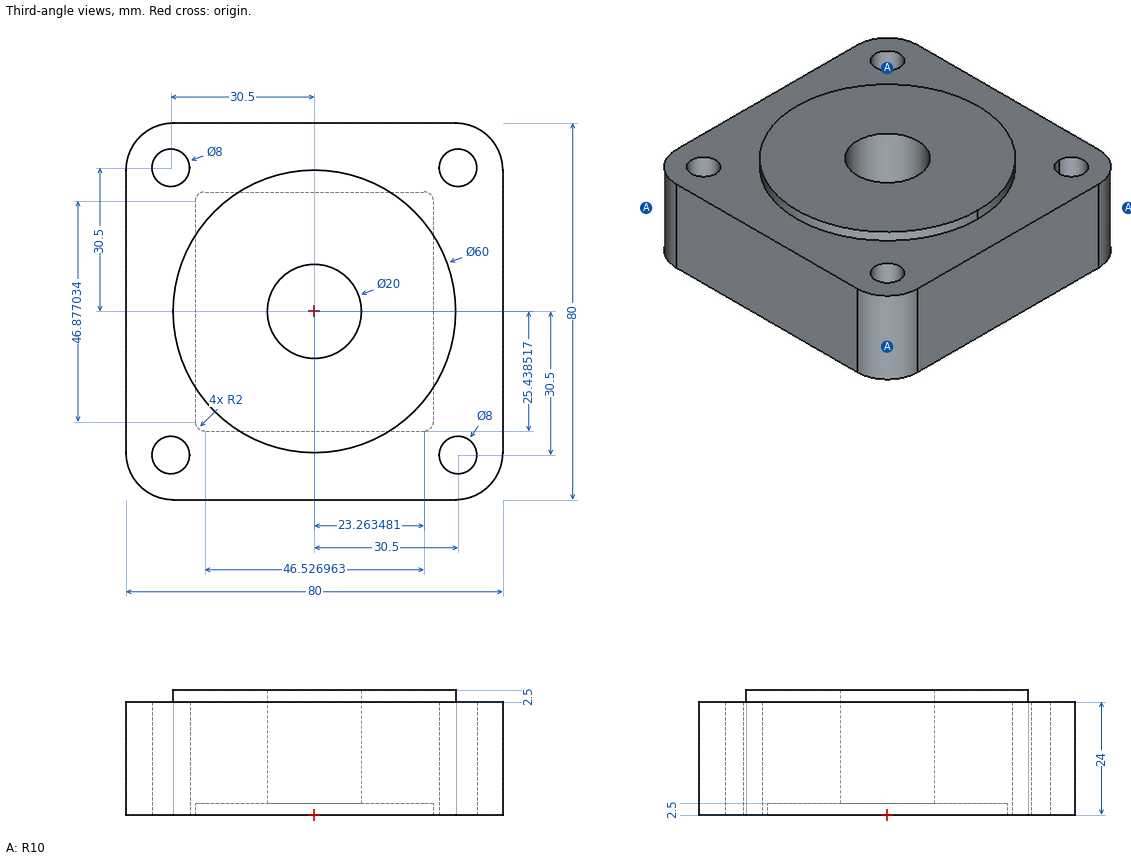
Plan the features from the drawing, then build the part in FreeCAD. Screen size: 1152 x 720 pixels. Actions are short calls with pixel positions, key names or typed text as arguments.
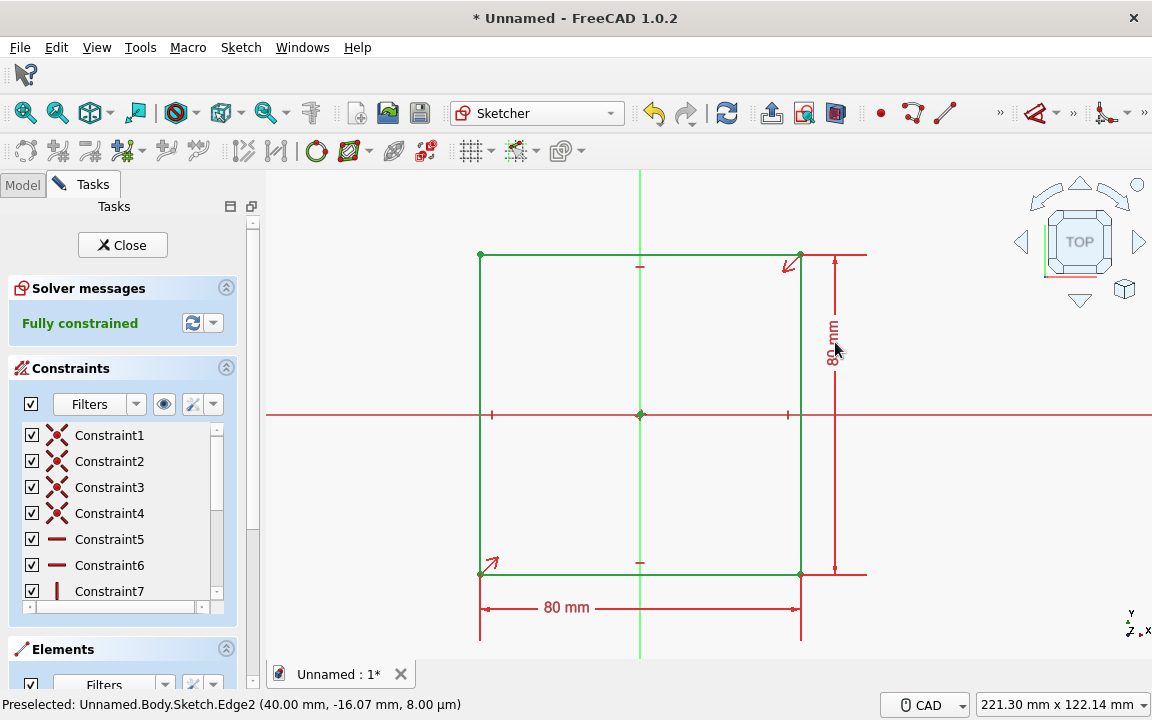
click(123, 245)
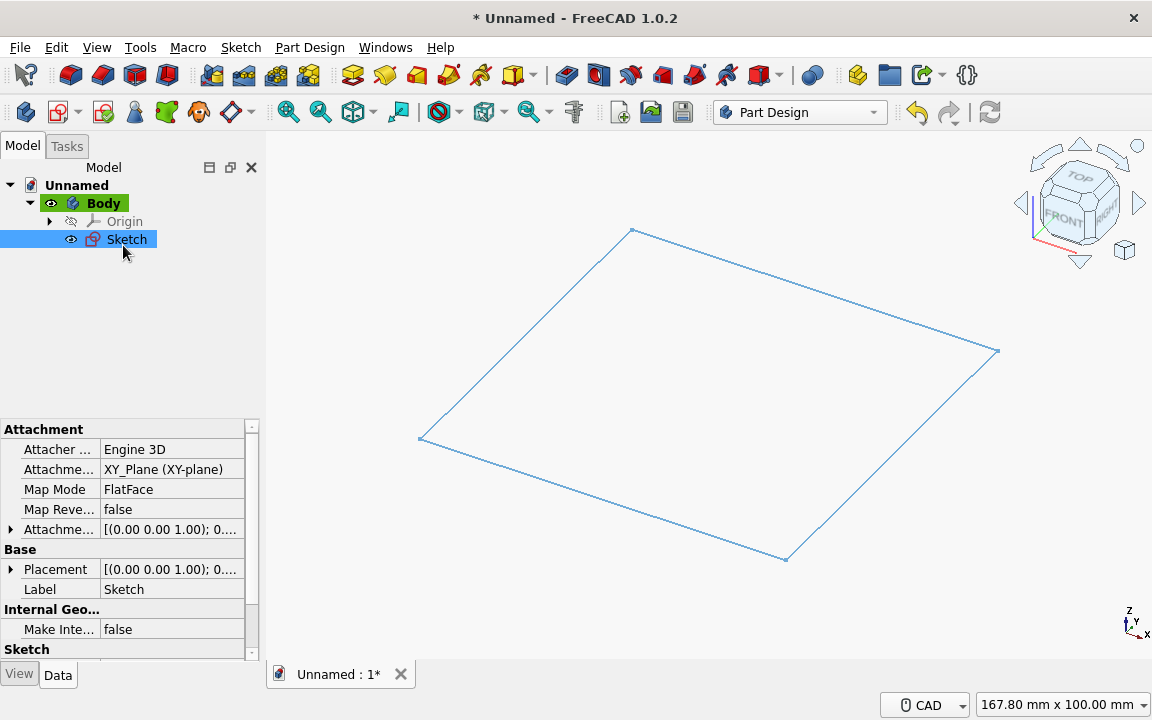
click(354, 76)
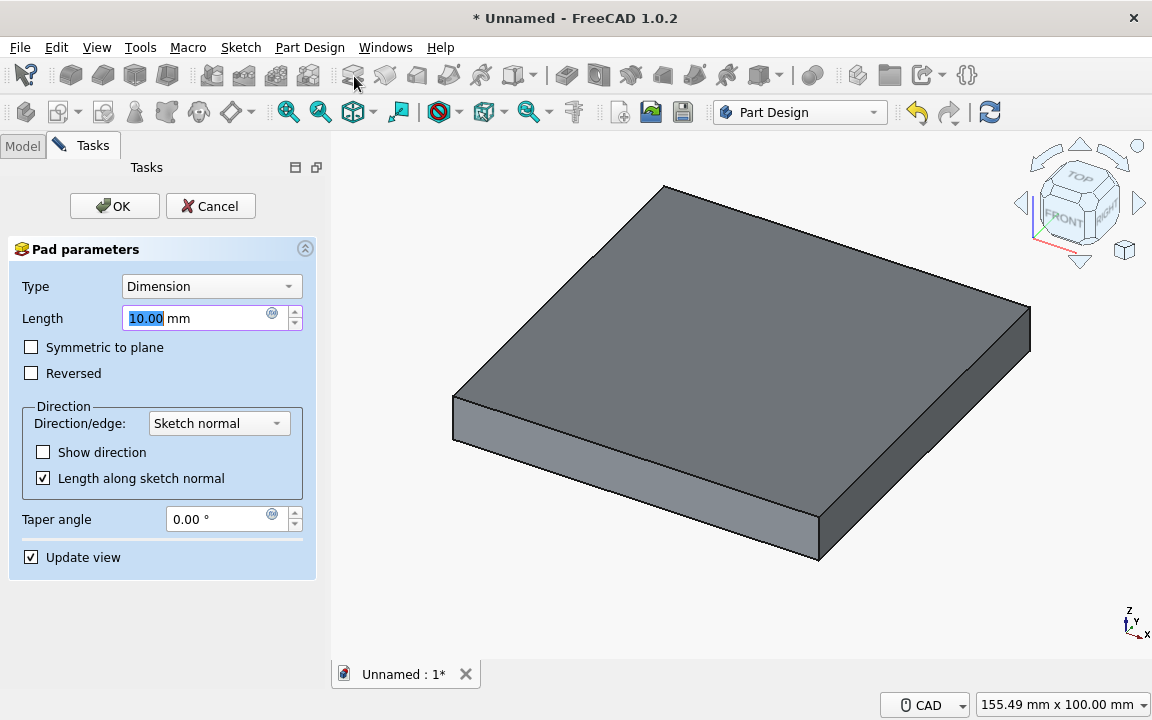
text(24)
key(Tab)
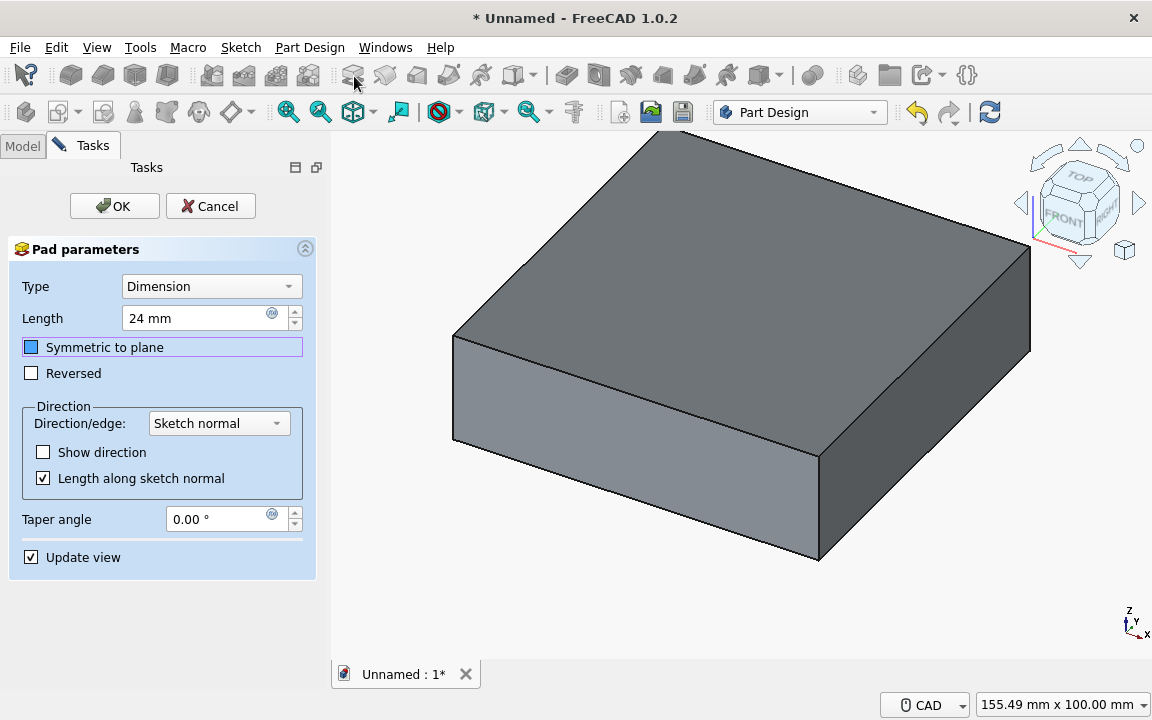
click(115, 206)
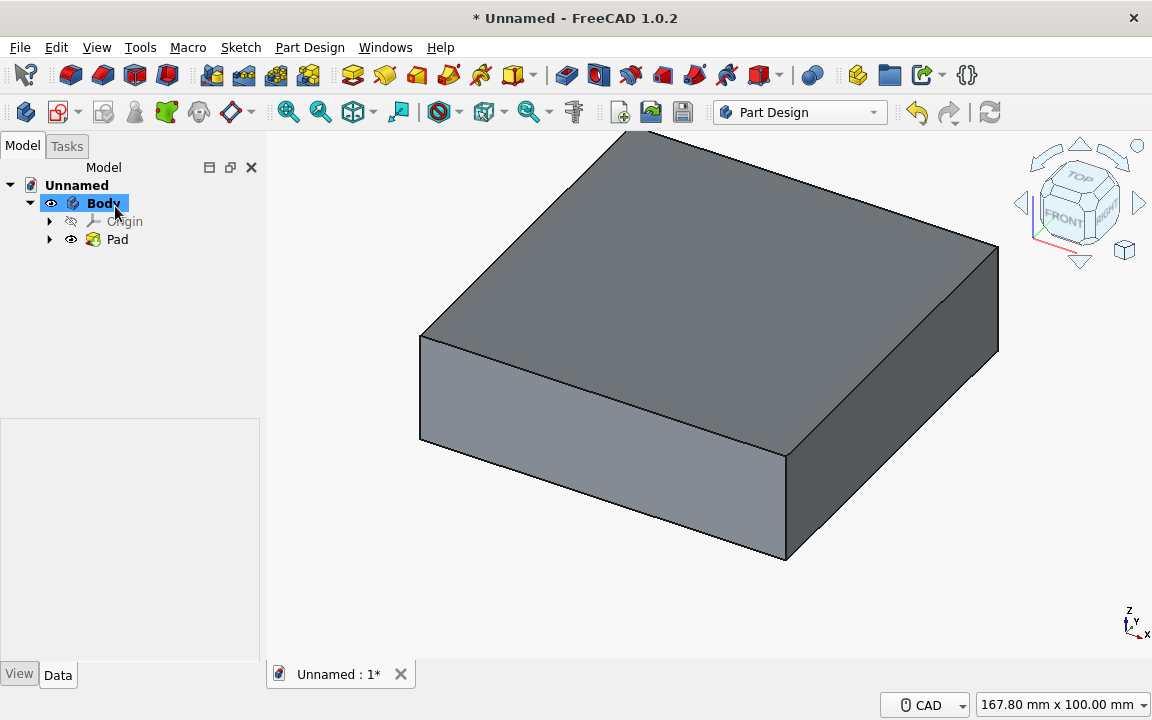
click(290, 112)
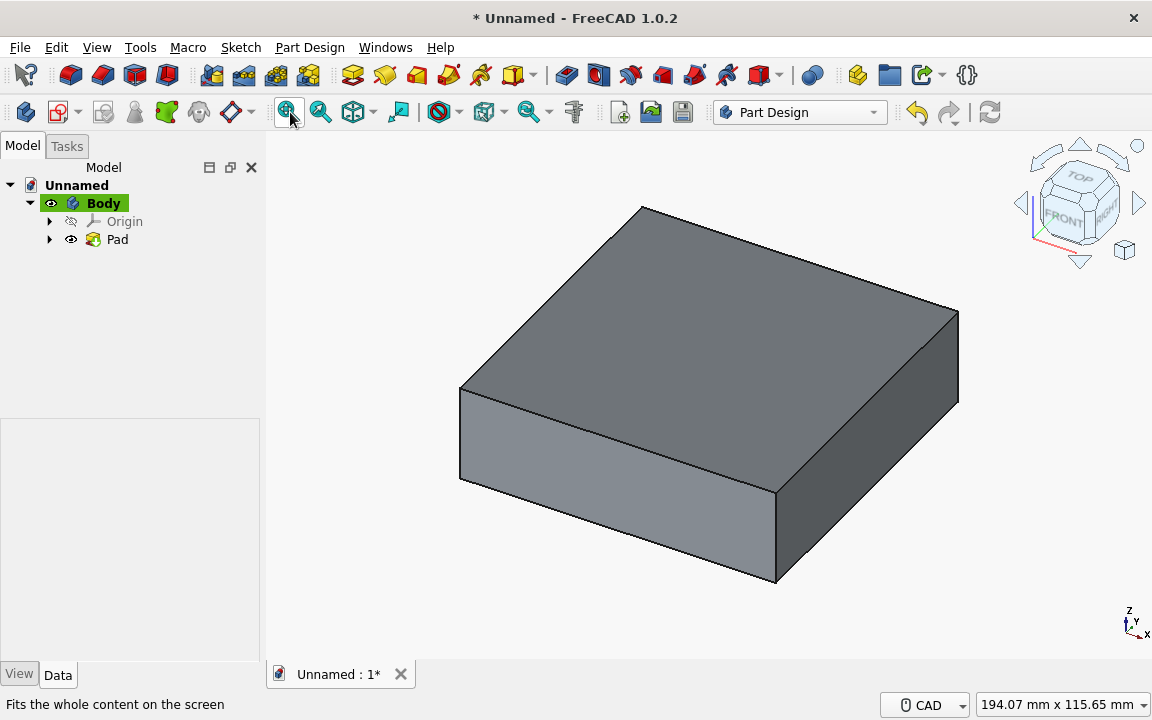
click(776, 537)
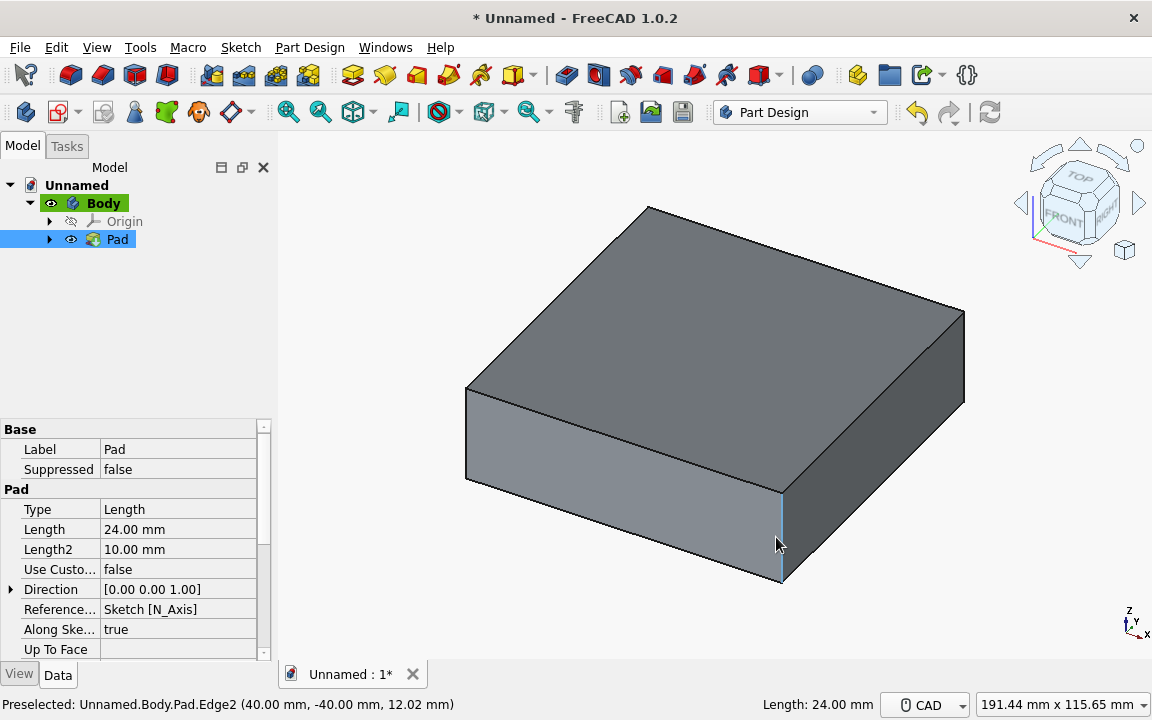
key(0)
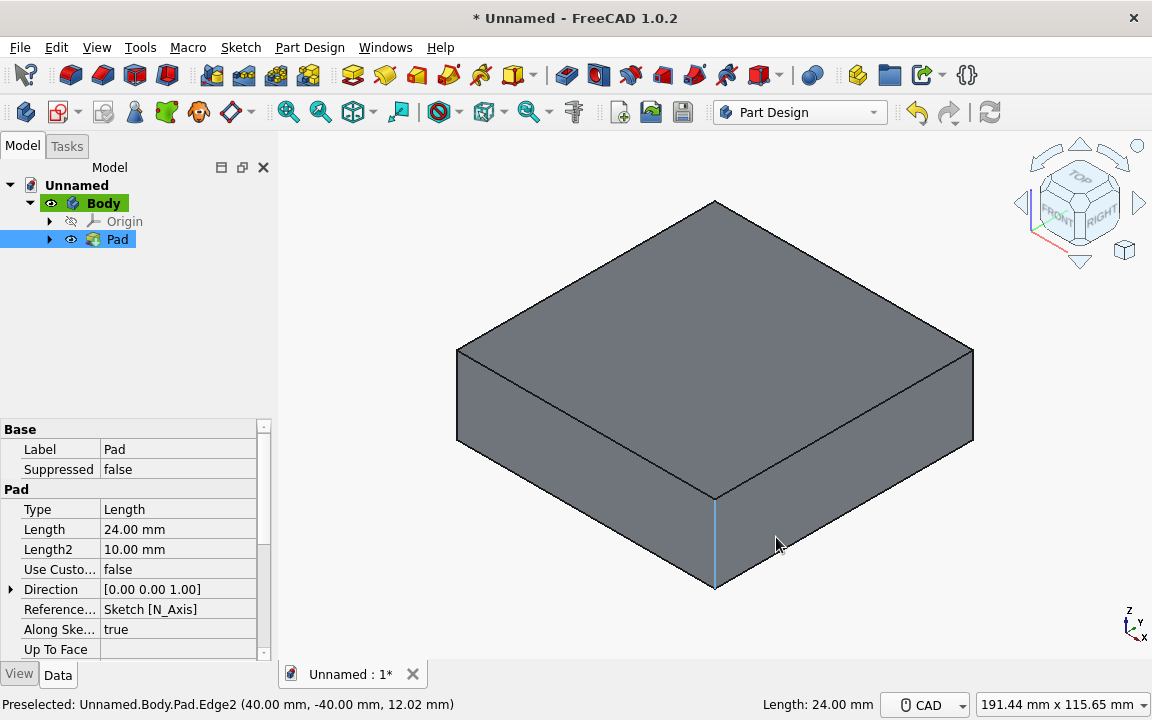
key(2)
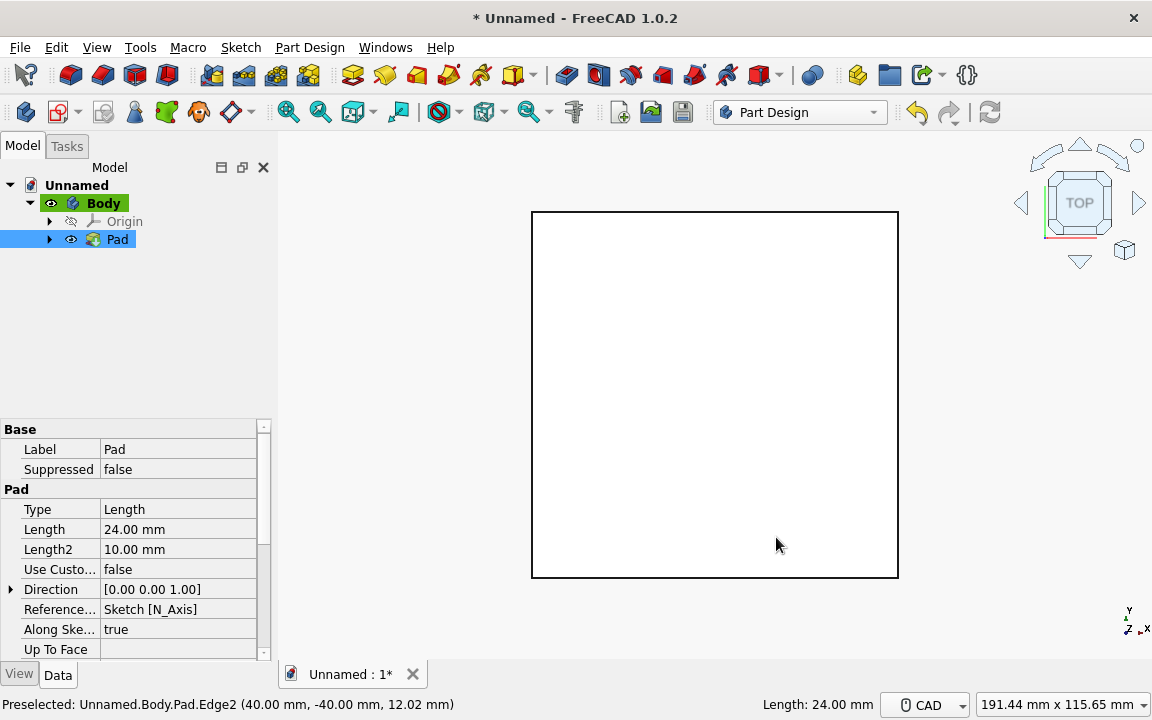
key(1)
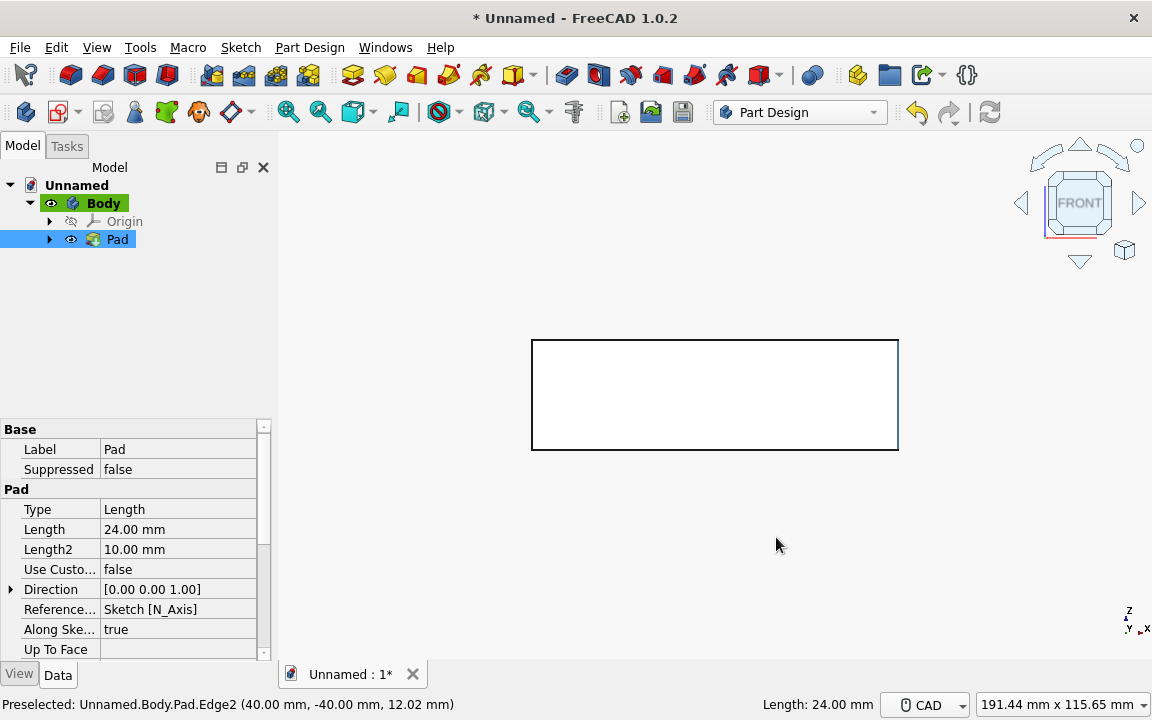
click(290, 112)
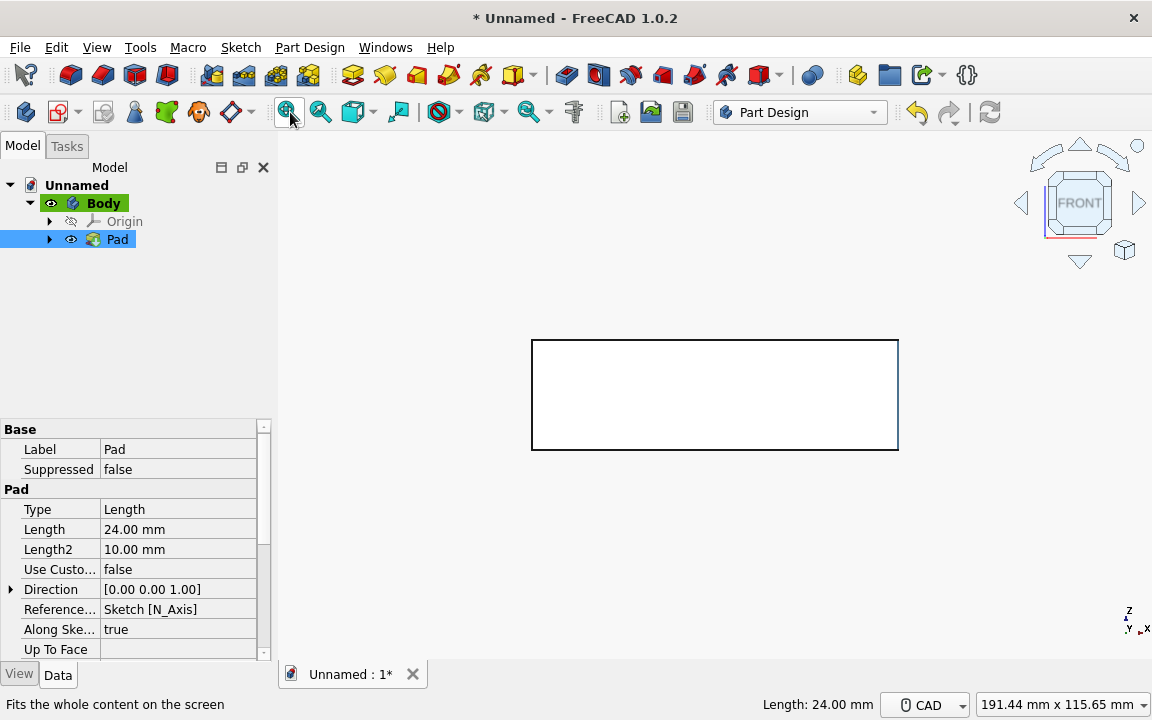
click(532, 394, ctrl)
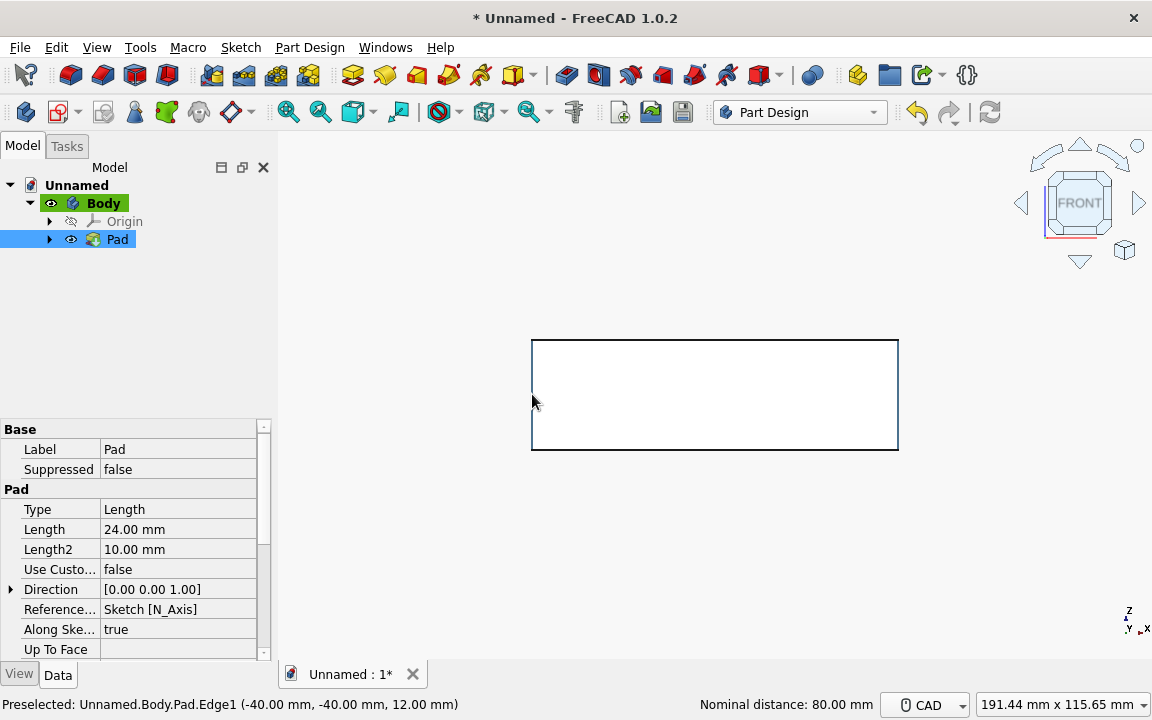
key(3)